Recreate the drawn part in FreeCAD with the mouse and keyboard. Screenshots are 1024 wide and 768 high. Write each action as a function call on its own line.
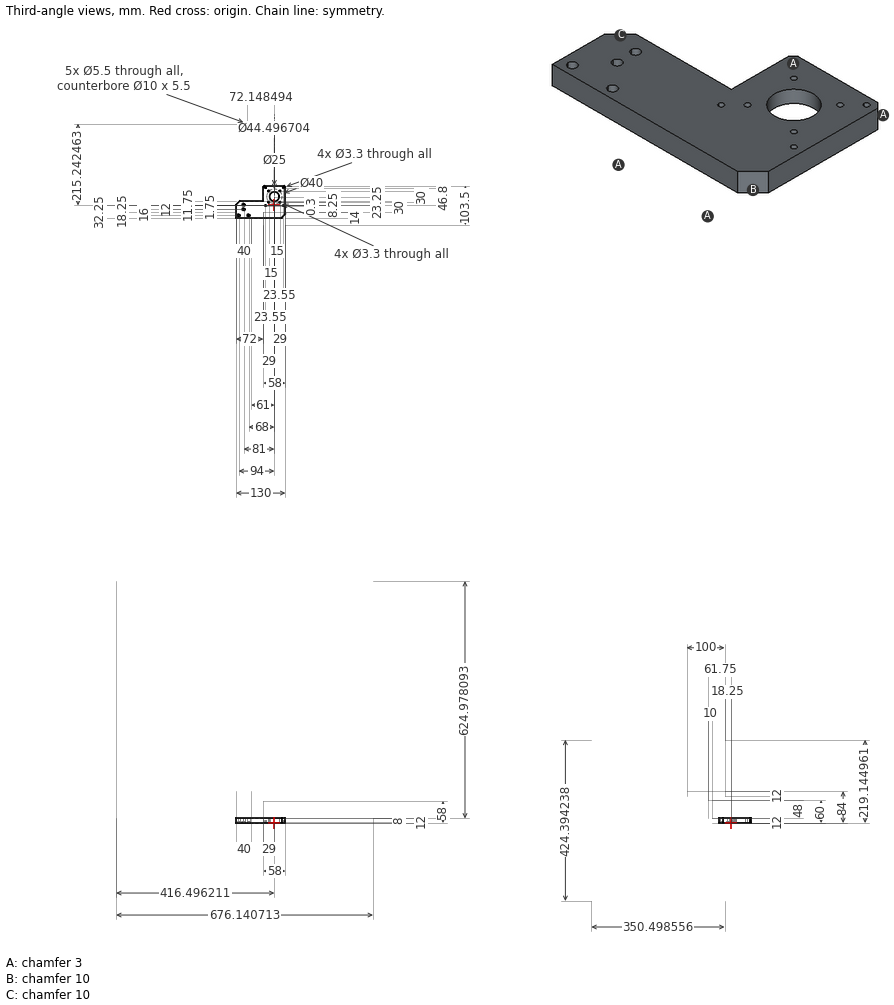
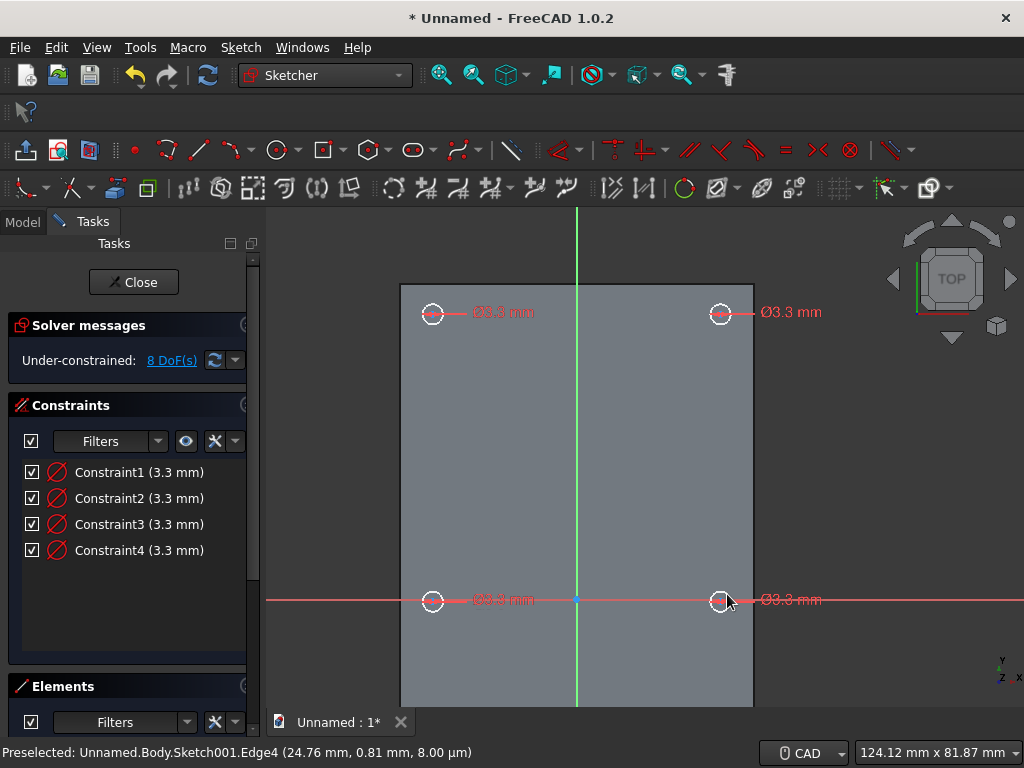
click(721, 314)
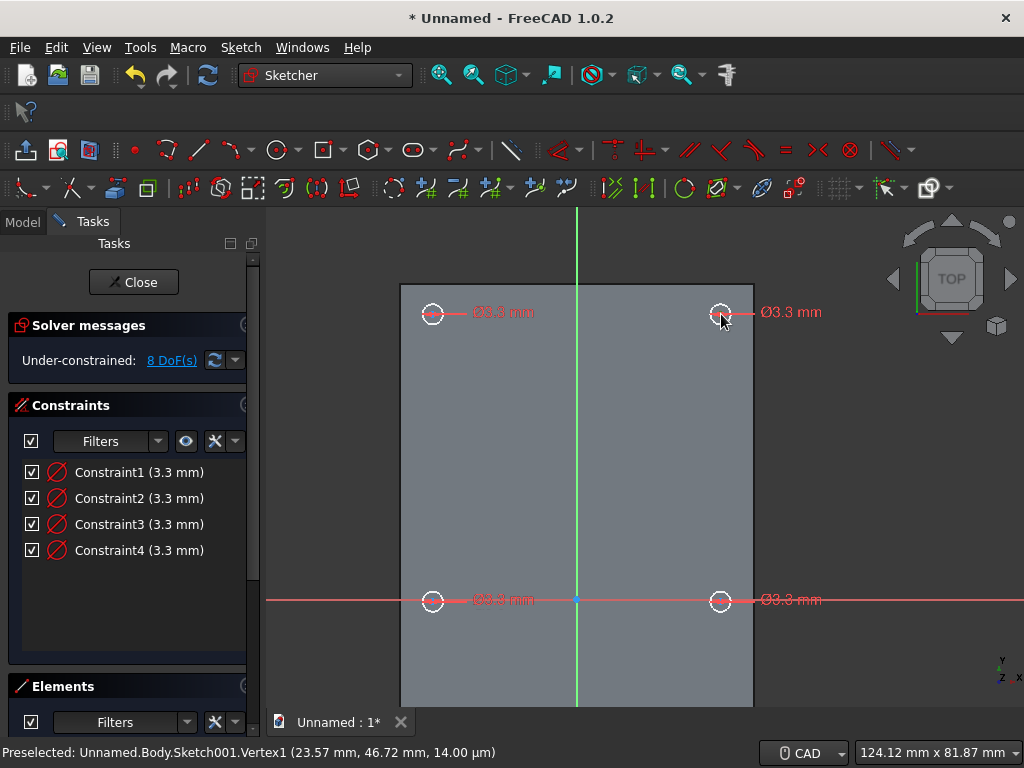
click(433, 314)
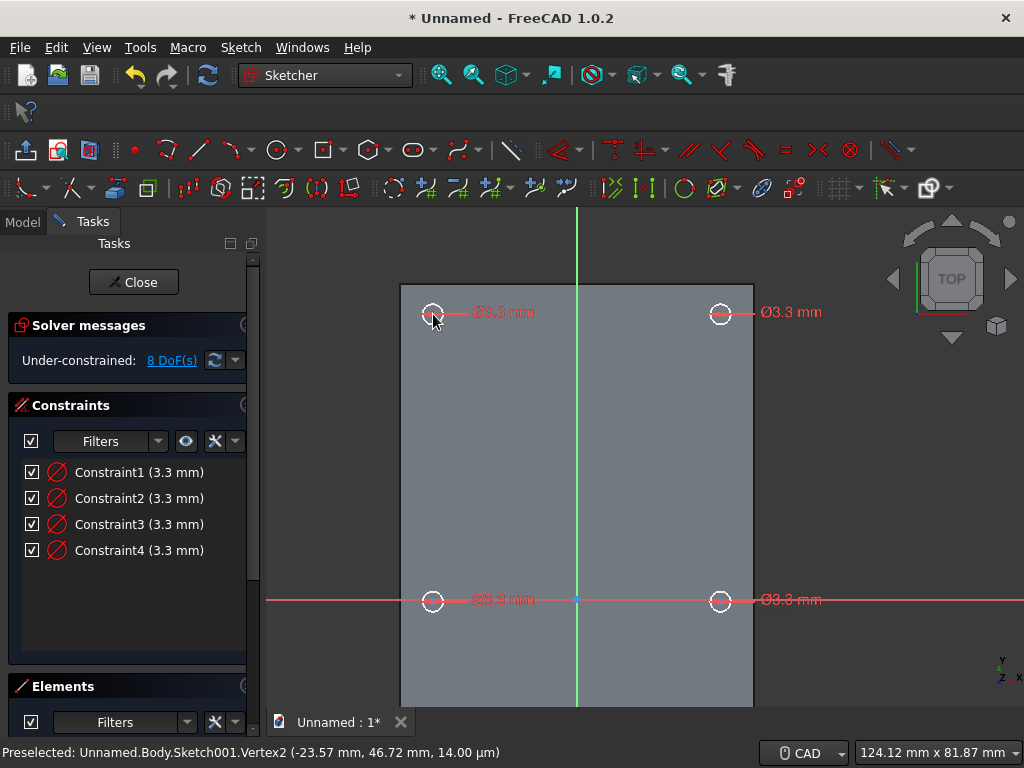
click(577, 647)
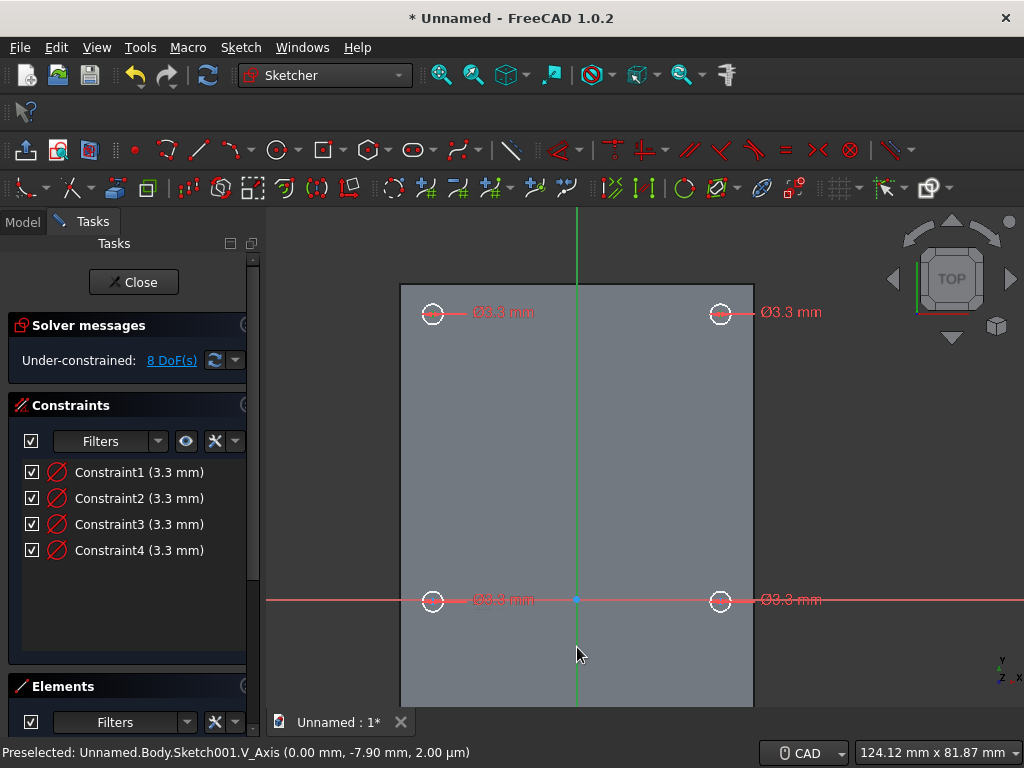
key(s)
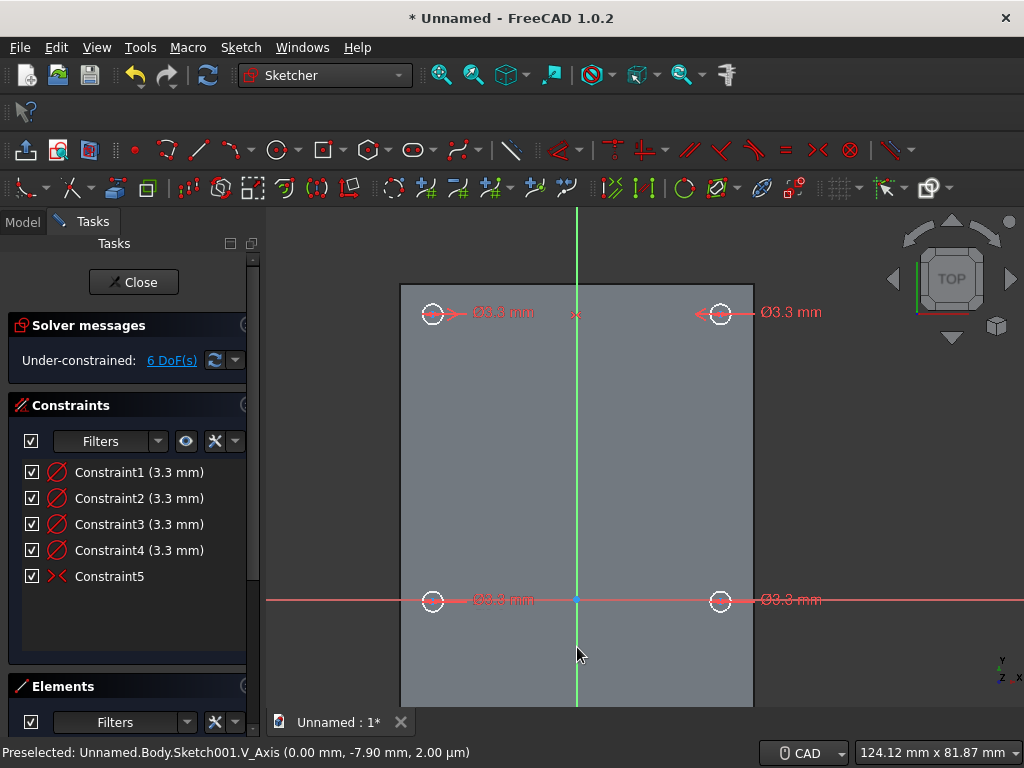
click(433, 602)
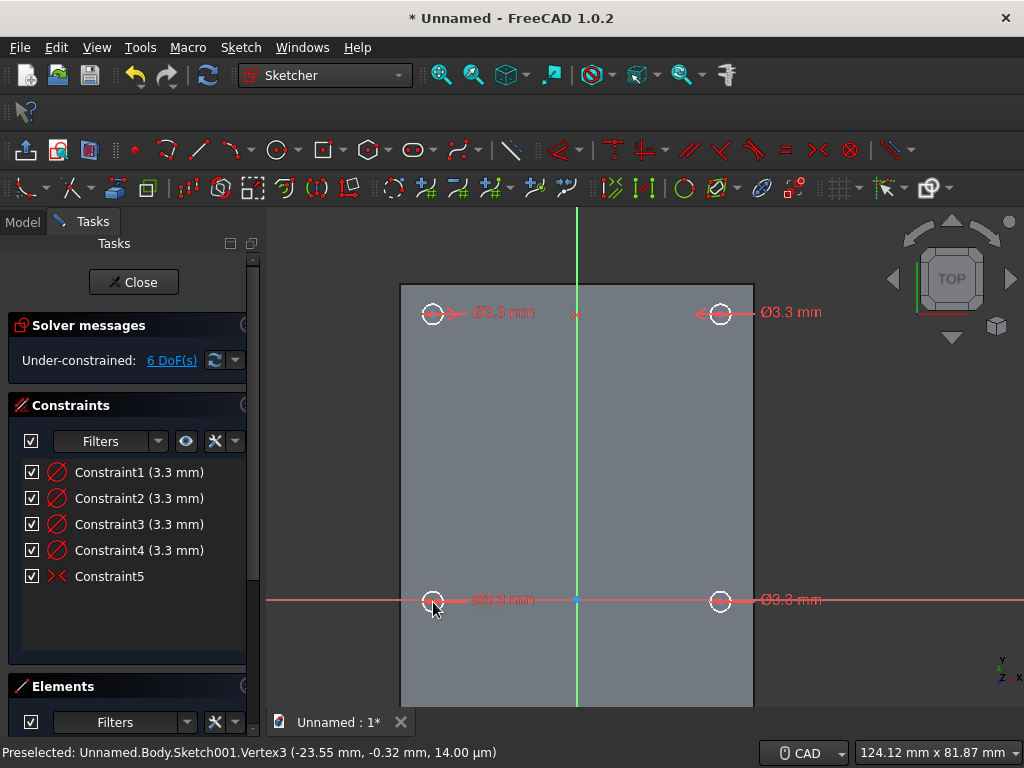
click(721, 602)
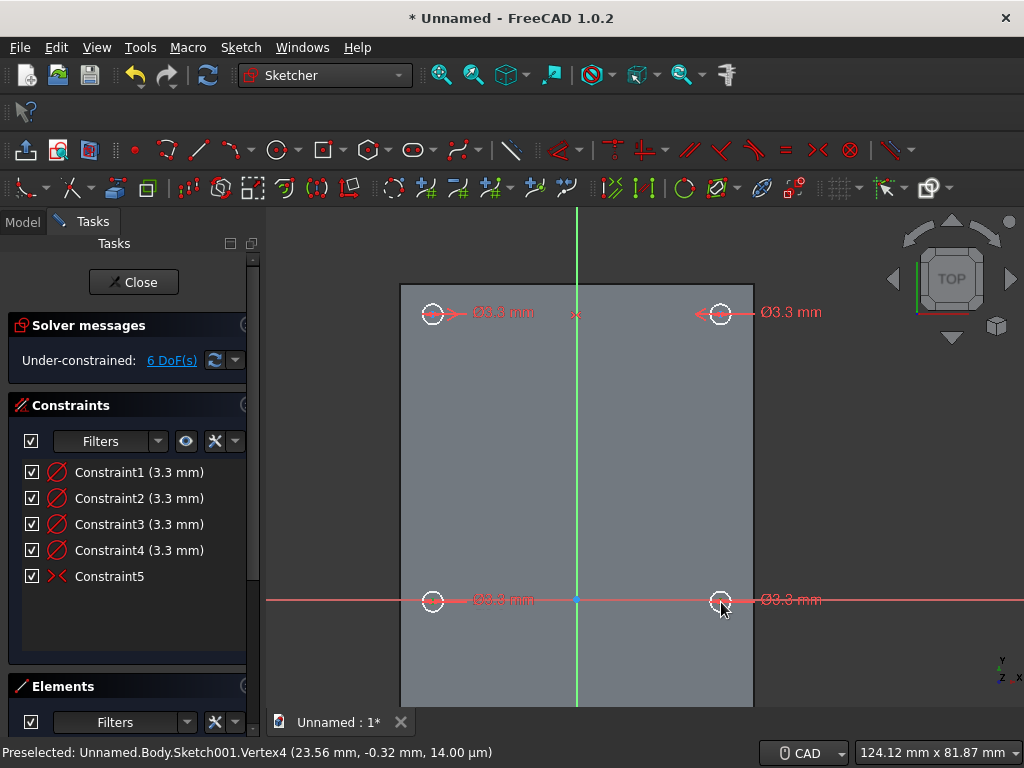
click(577, 647)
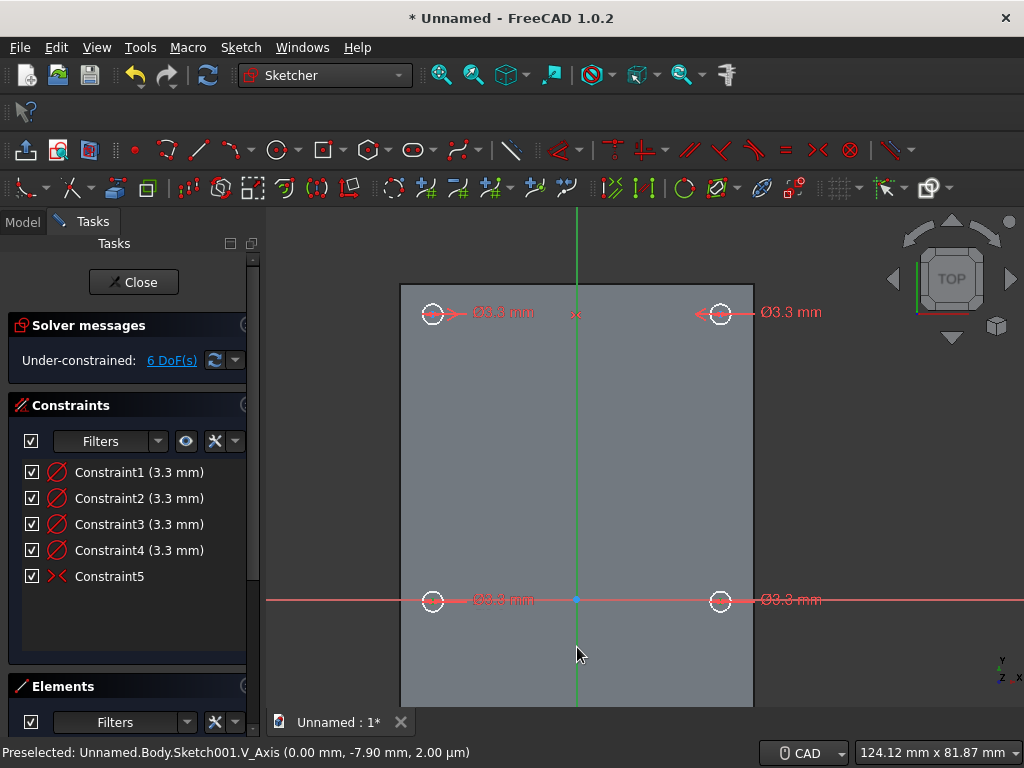
click(818, 150)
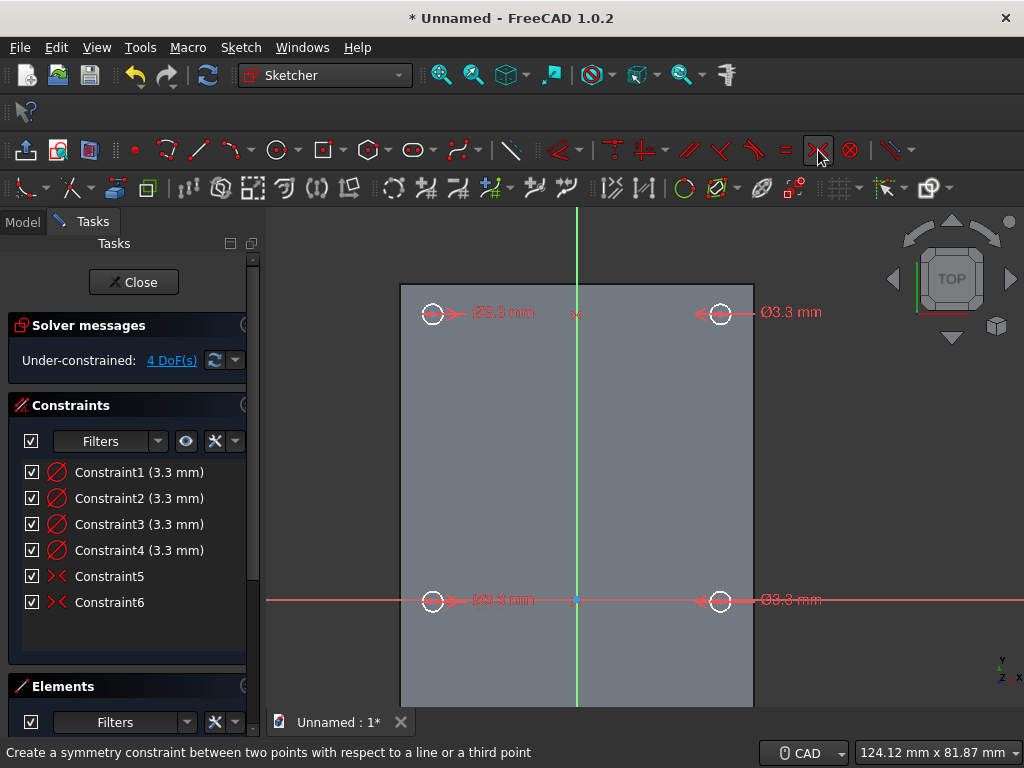
click(558, 150)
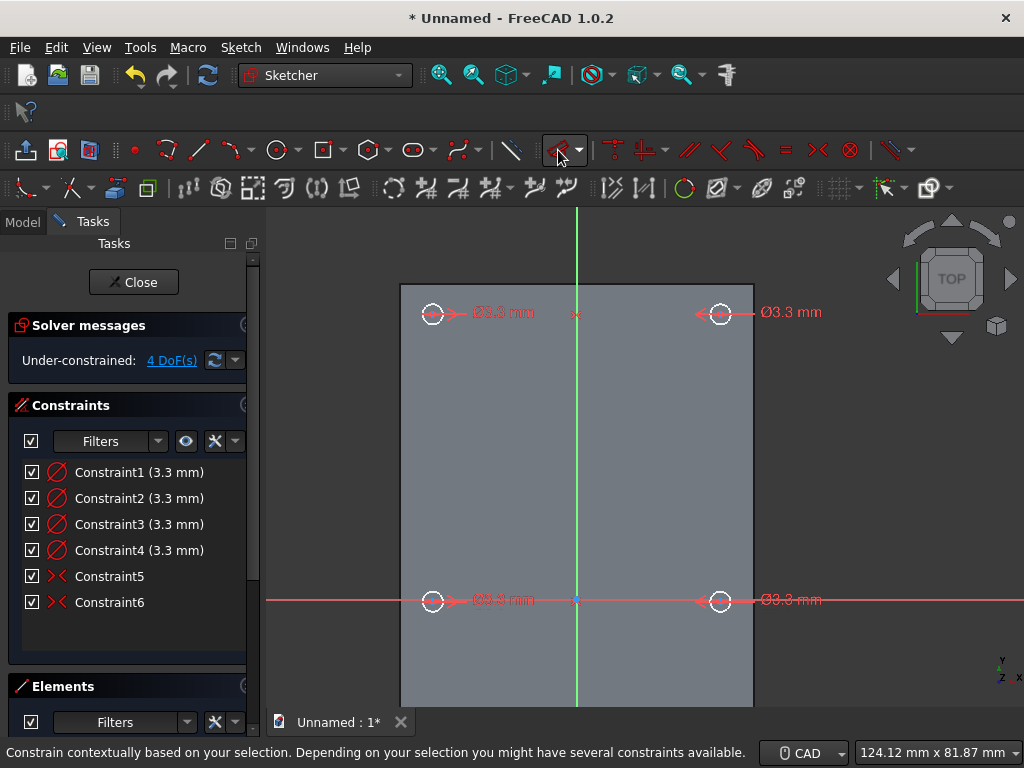
scroll(433, 602, up, 16)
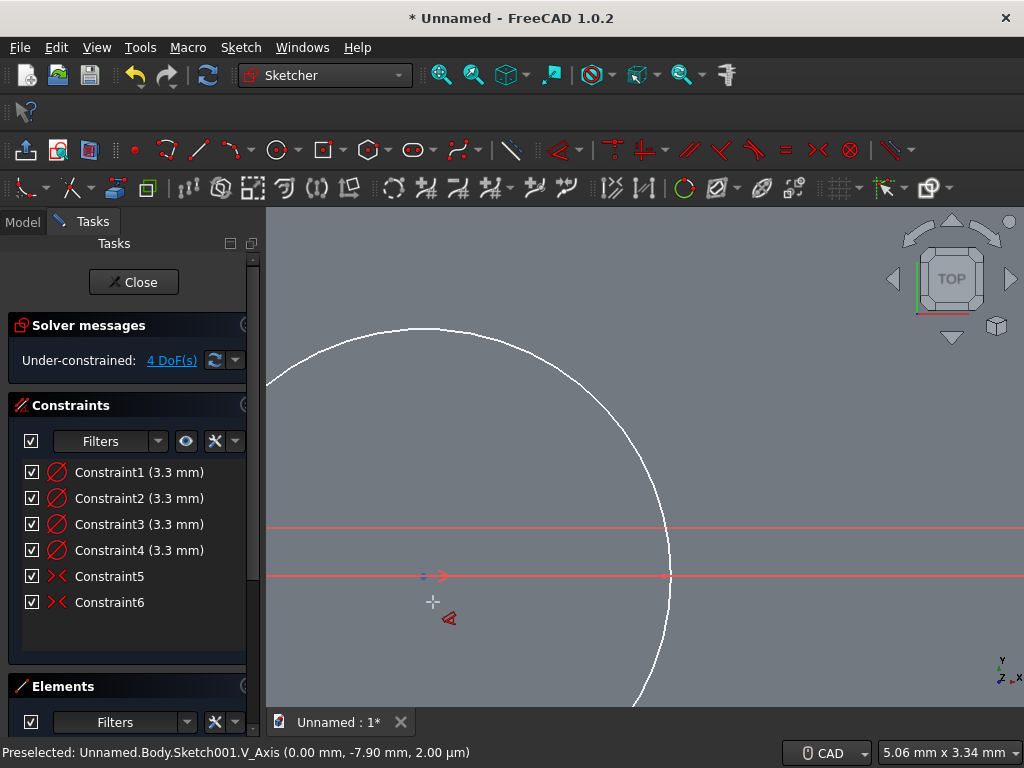
click(424, 576)
click(390, 552)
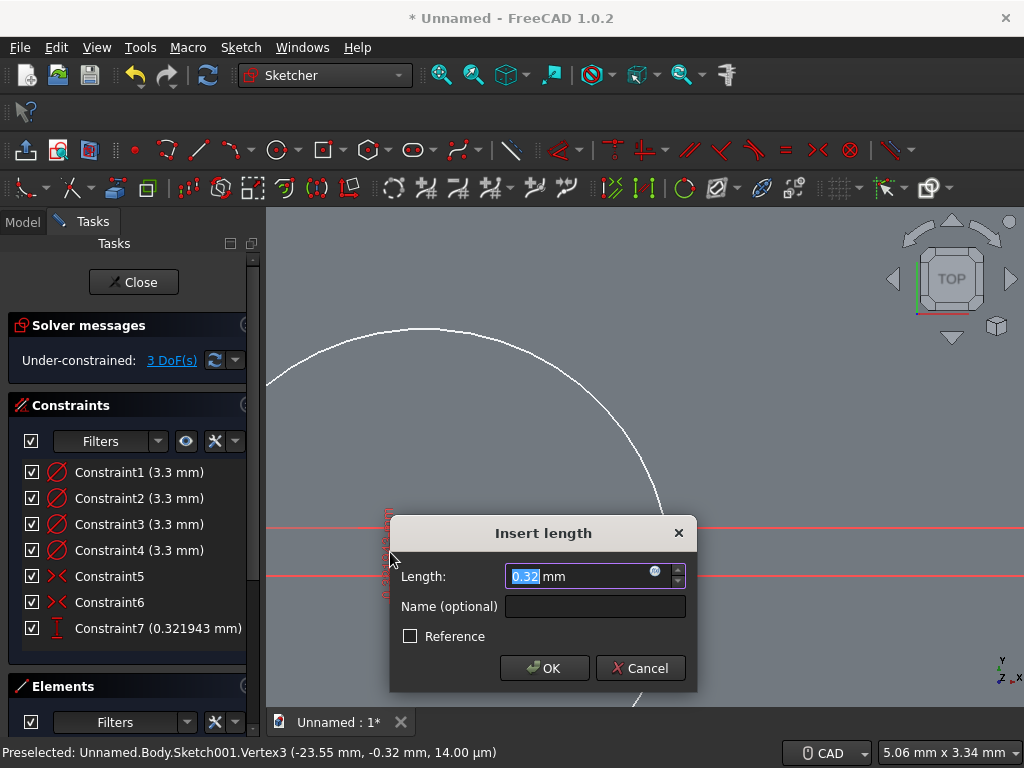
text(0.3)
key(Return)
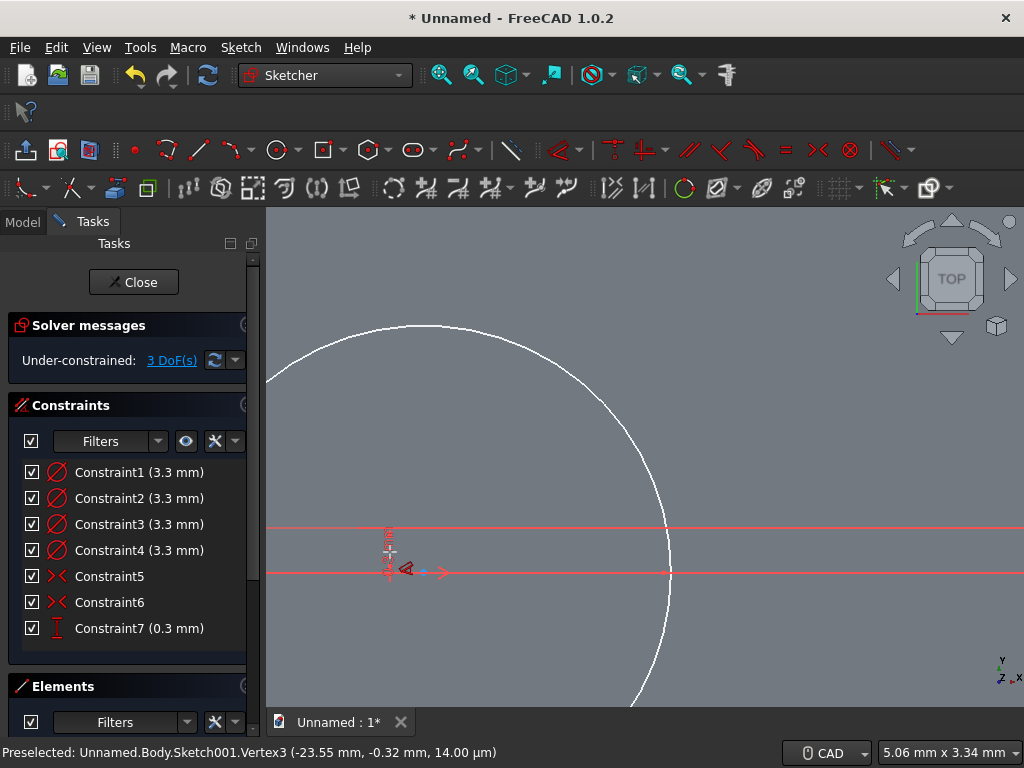
scroll(400, 636, down, 15)